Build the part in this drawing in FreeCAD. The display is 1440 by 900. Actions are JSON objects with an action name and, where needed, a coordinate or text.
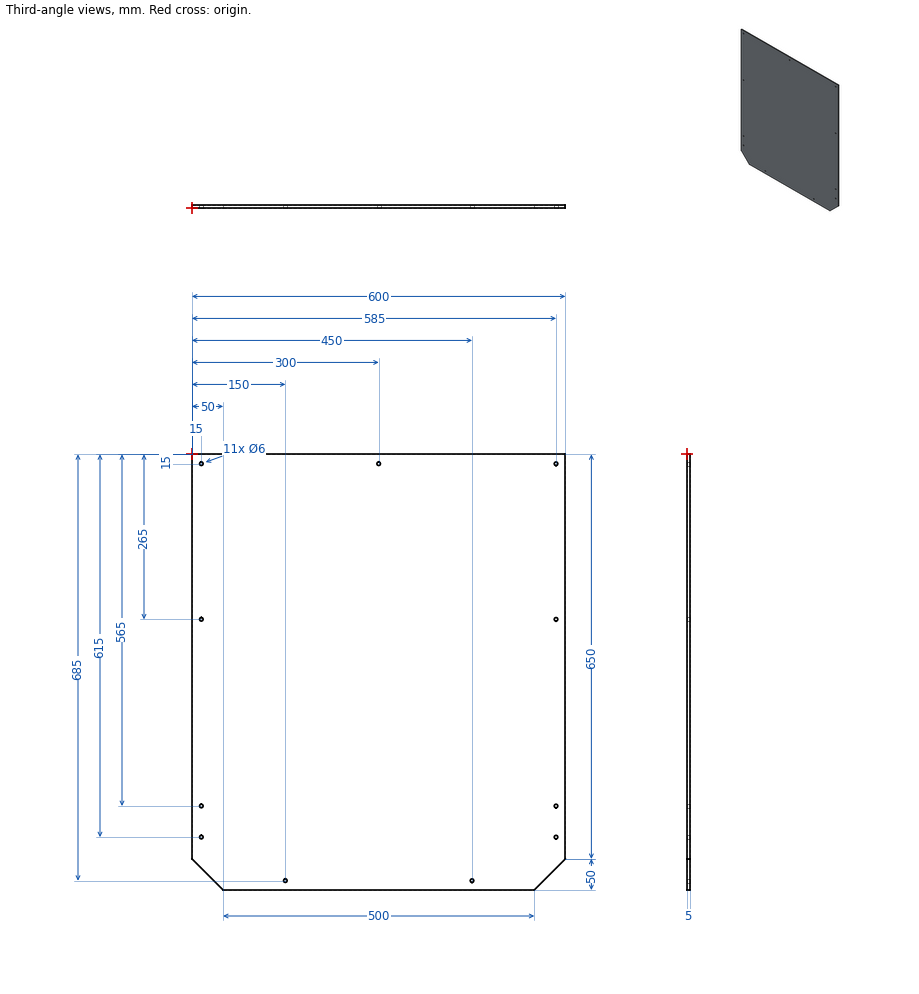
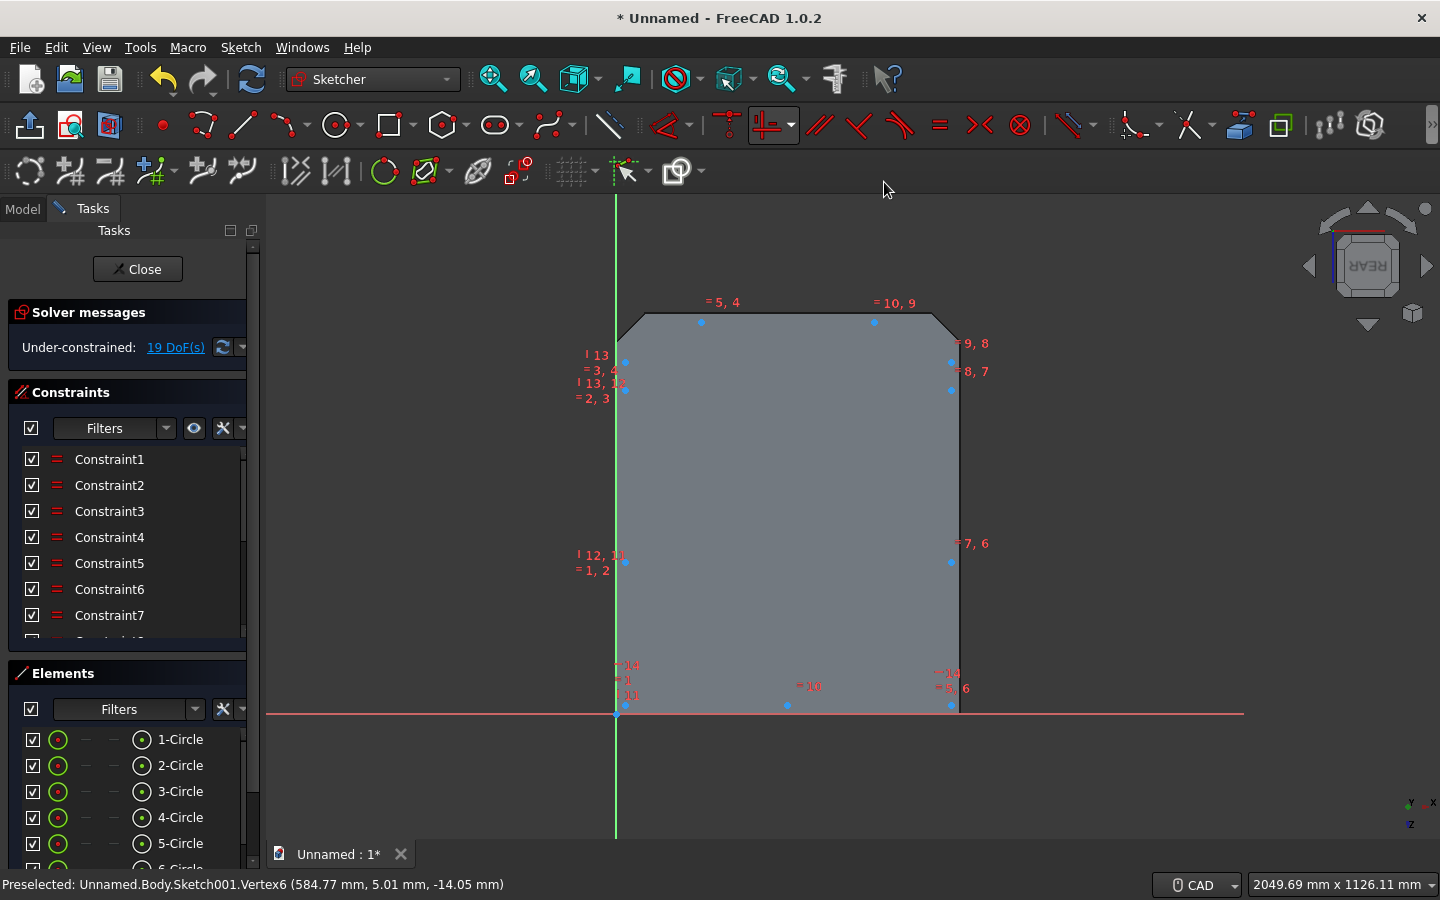
{"action": "left_click", "coordinate": [951, 706]}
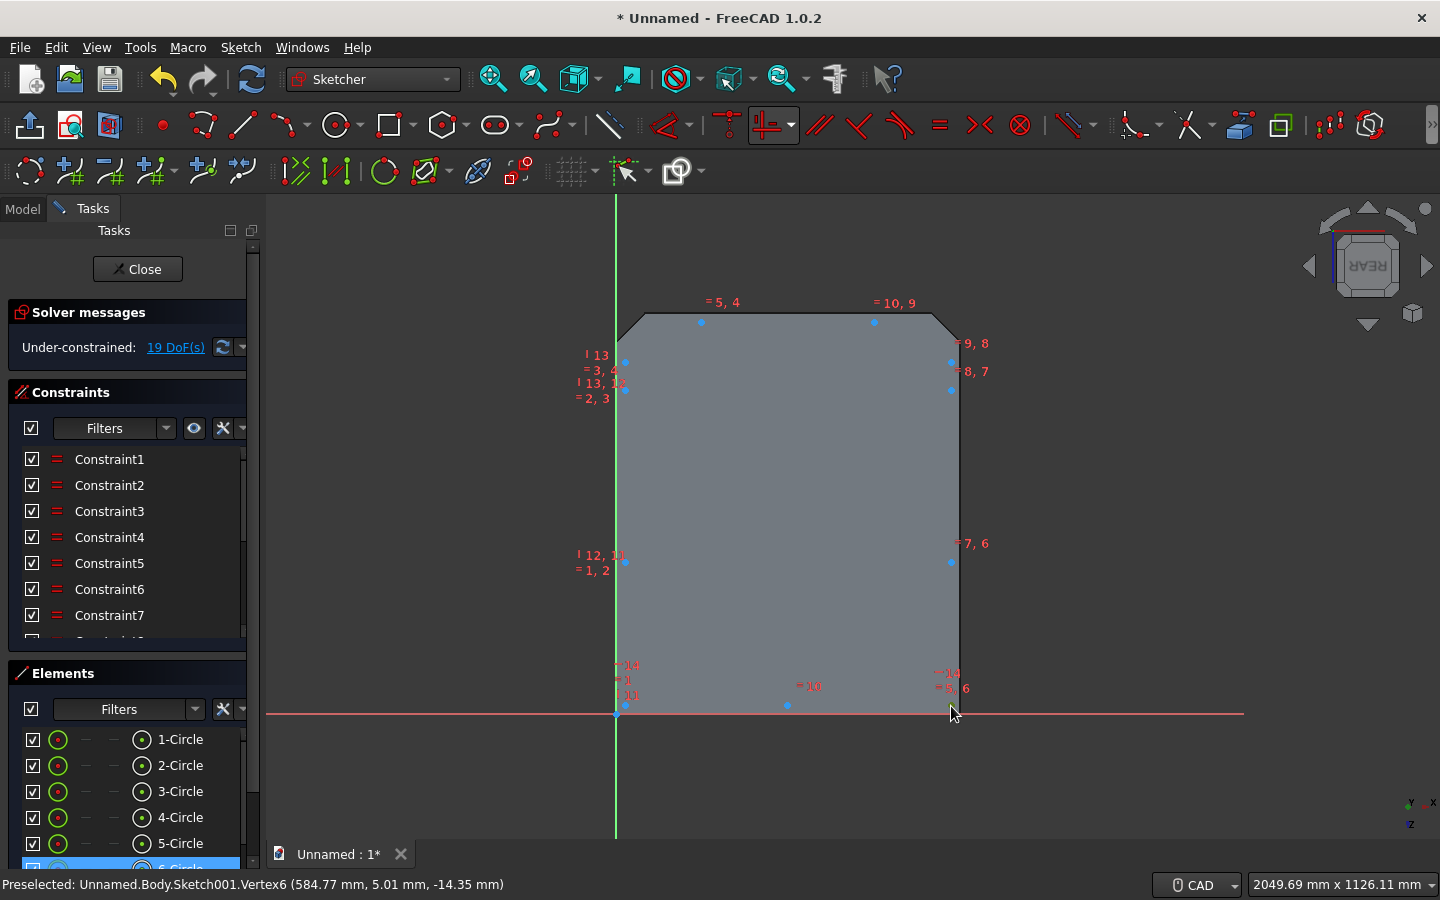
{"action": "left_click", "coordinate": [951, 563]}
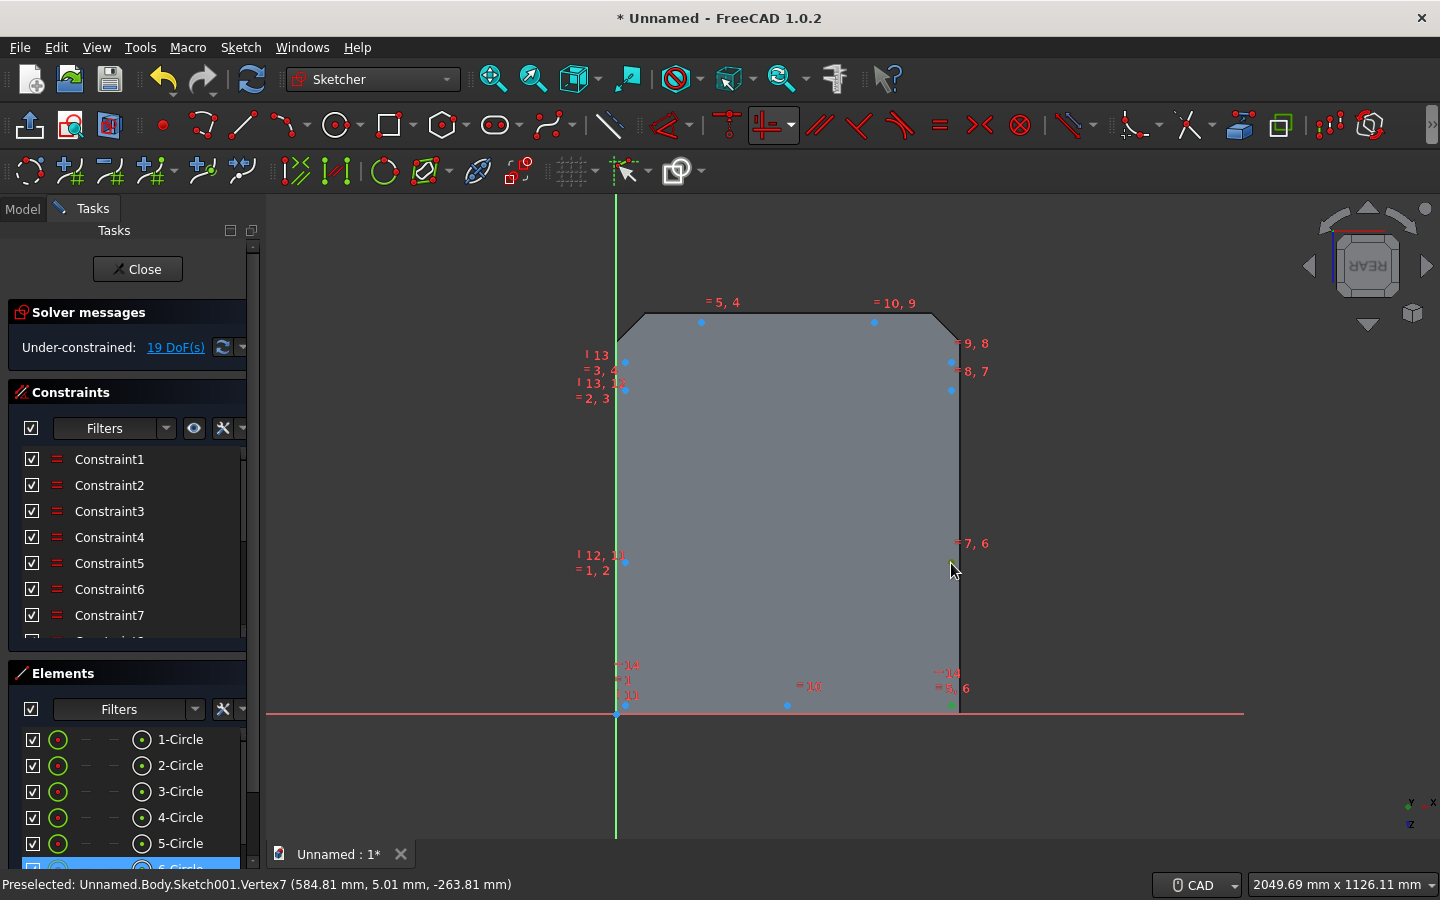
{"action": "key", "text": "v"}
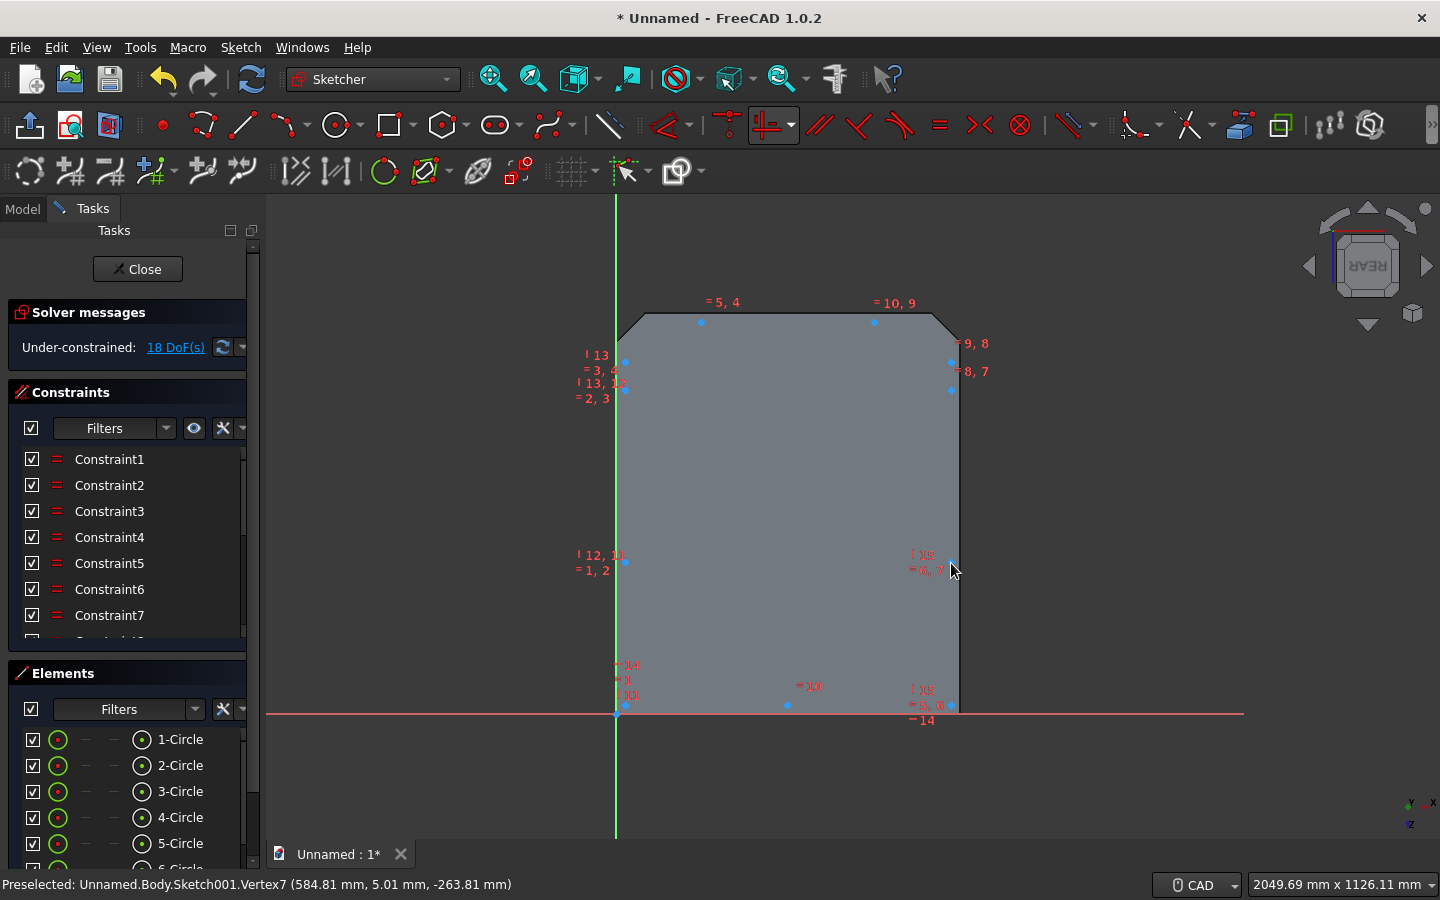
{"action": "left_click", "coordinate": [625, 563]}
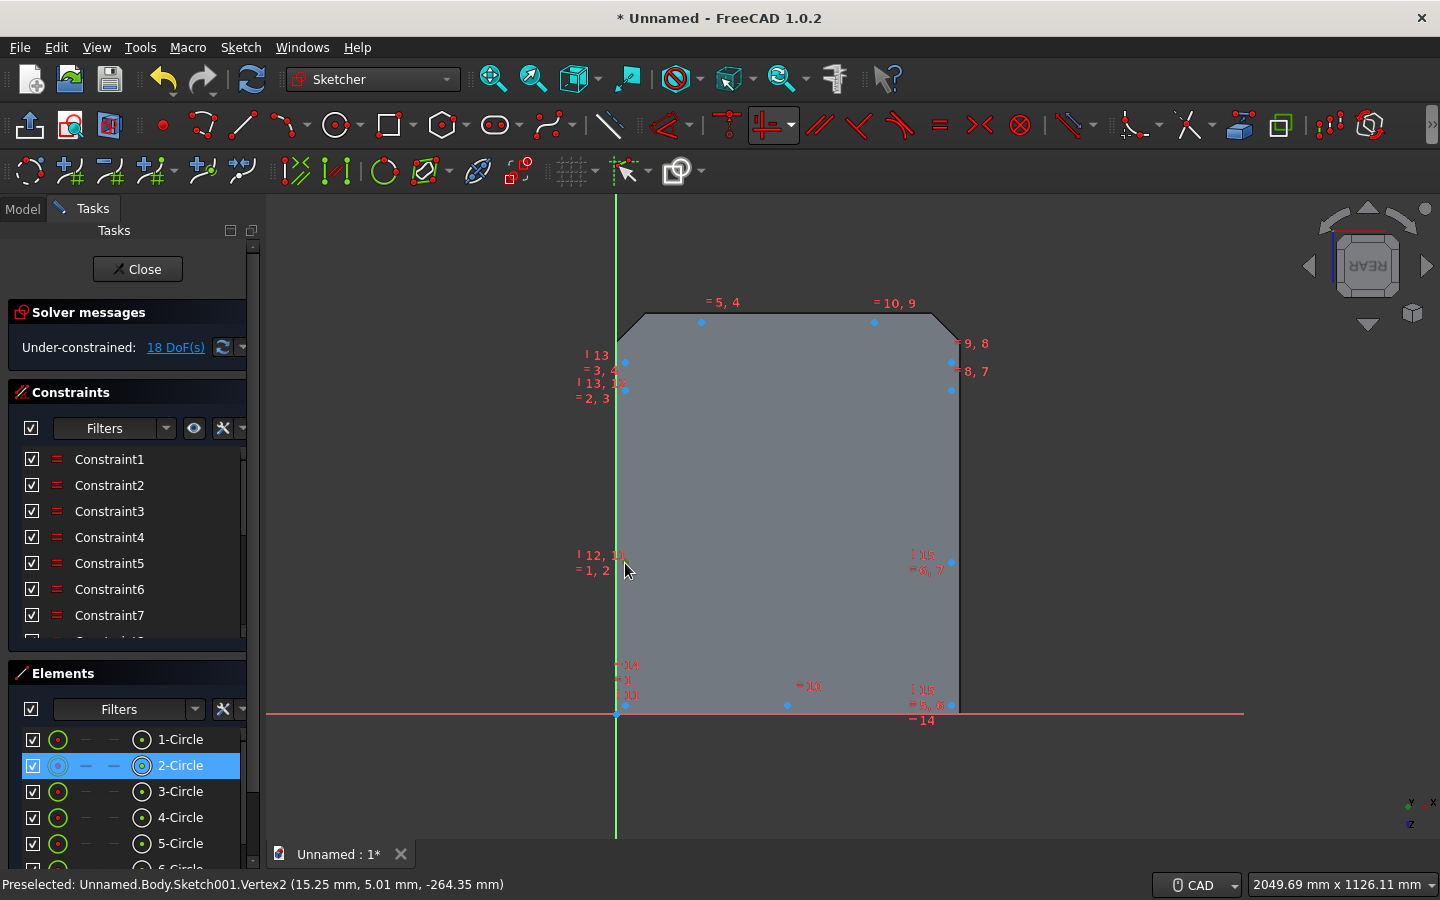
{"action": "left_click", "coordinate": [951, 563]}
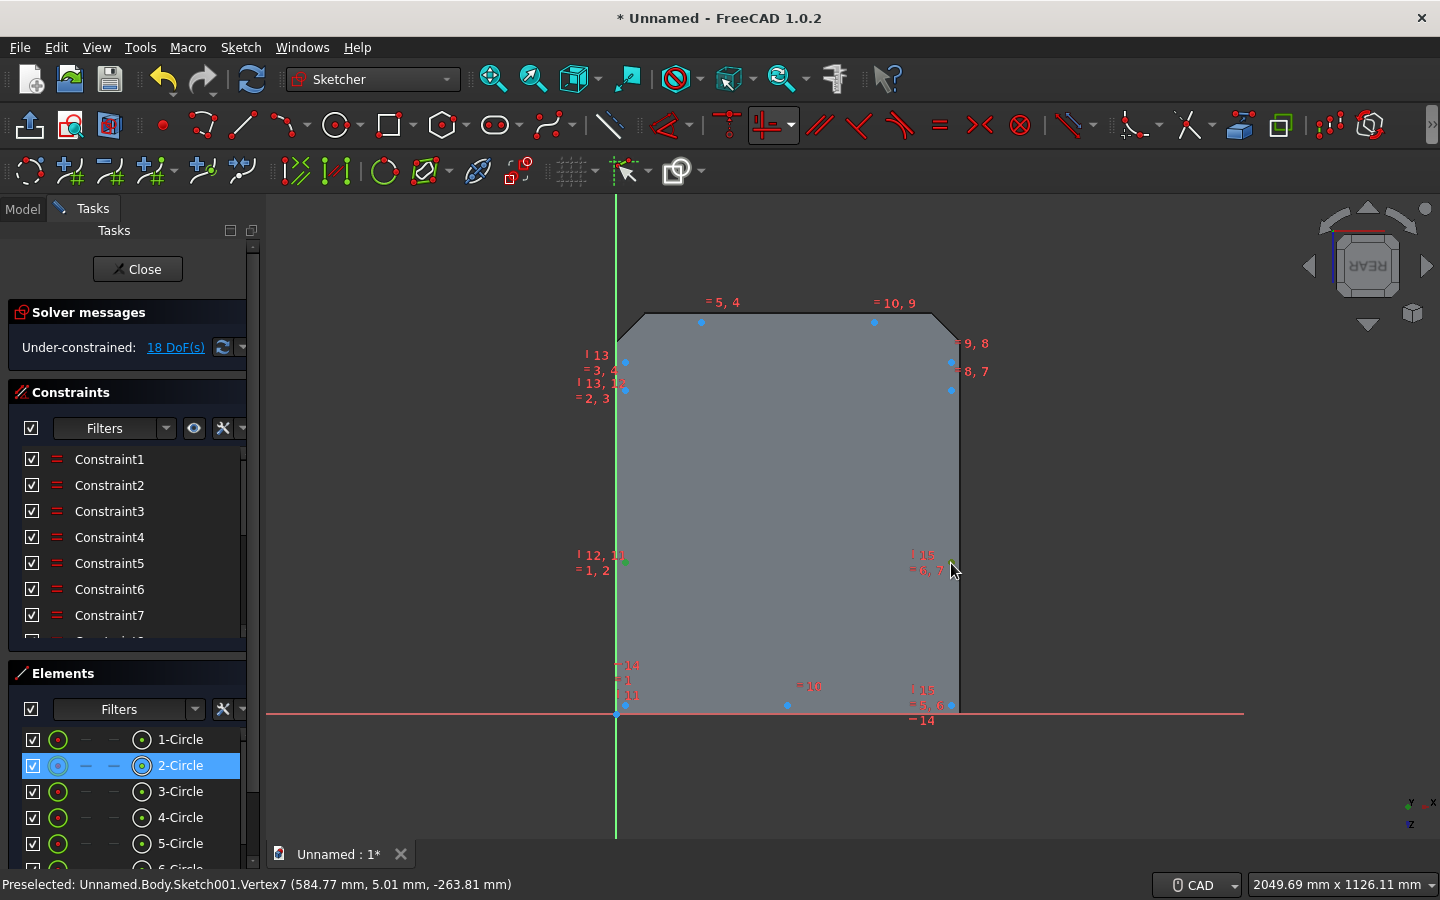
{"action": "key", "text": "h"}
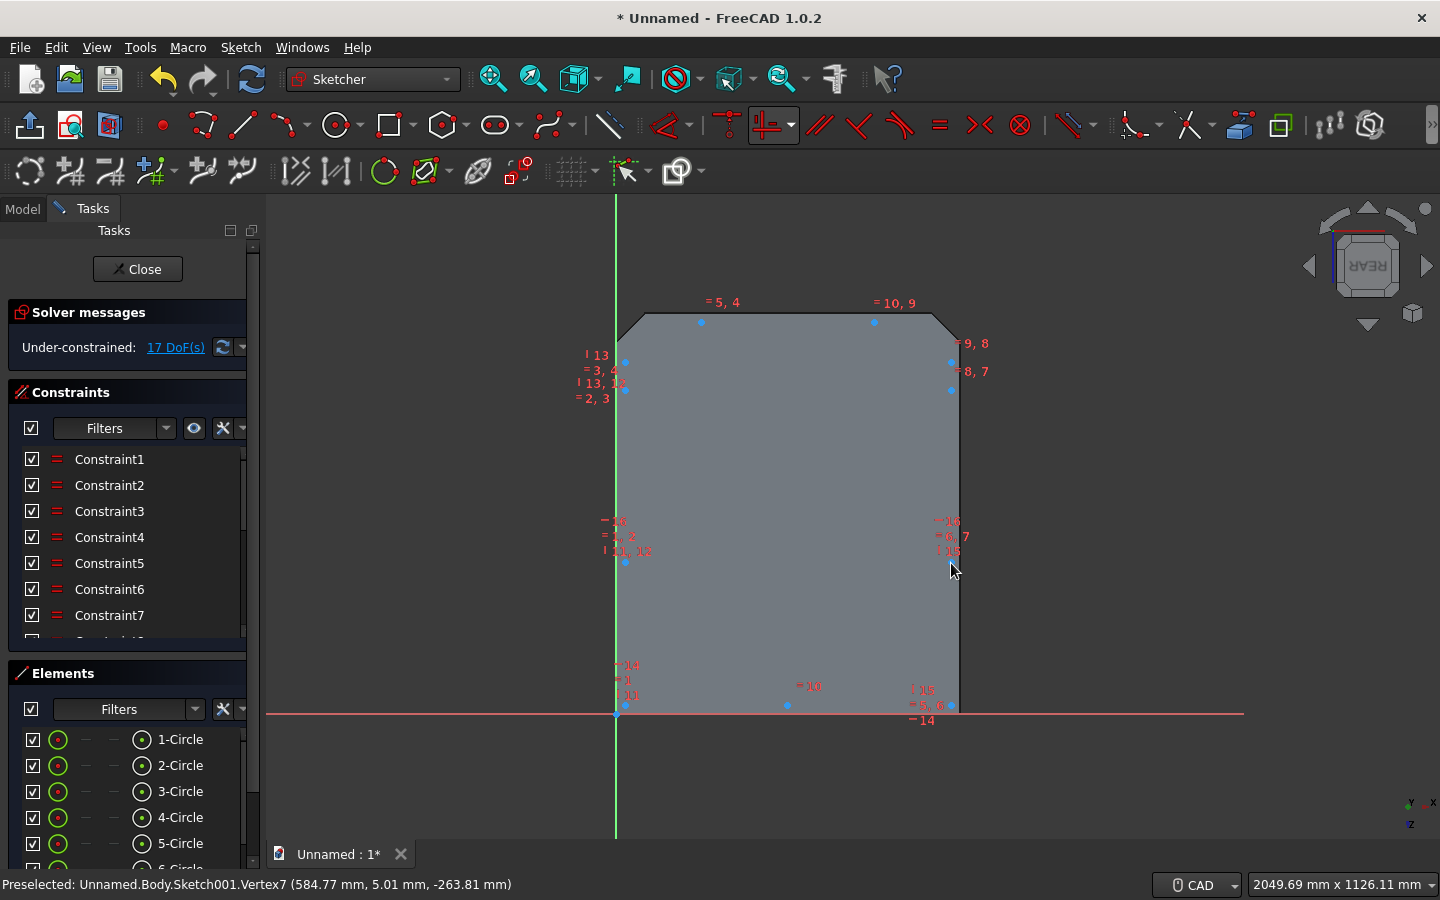
{"action": "left_click", "coordinate": [951, 563]}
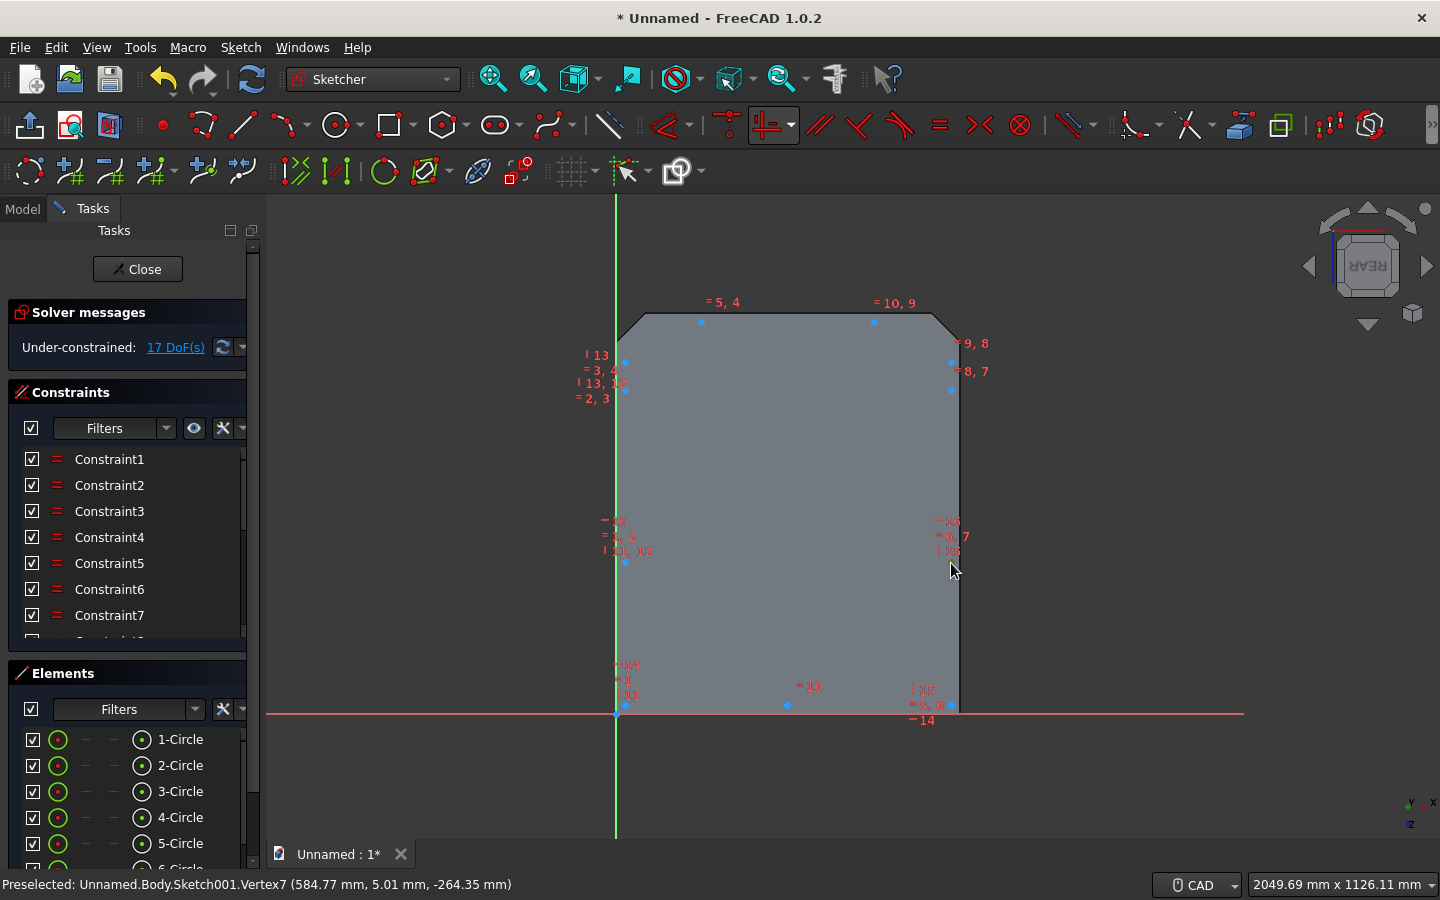
{"action": "left_click", "coordinate": [951, 391]}